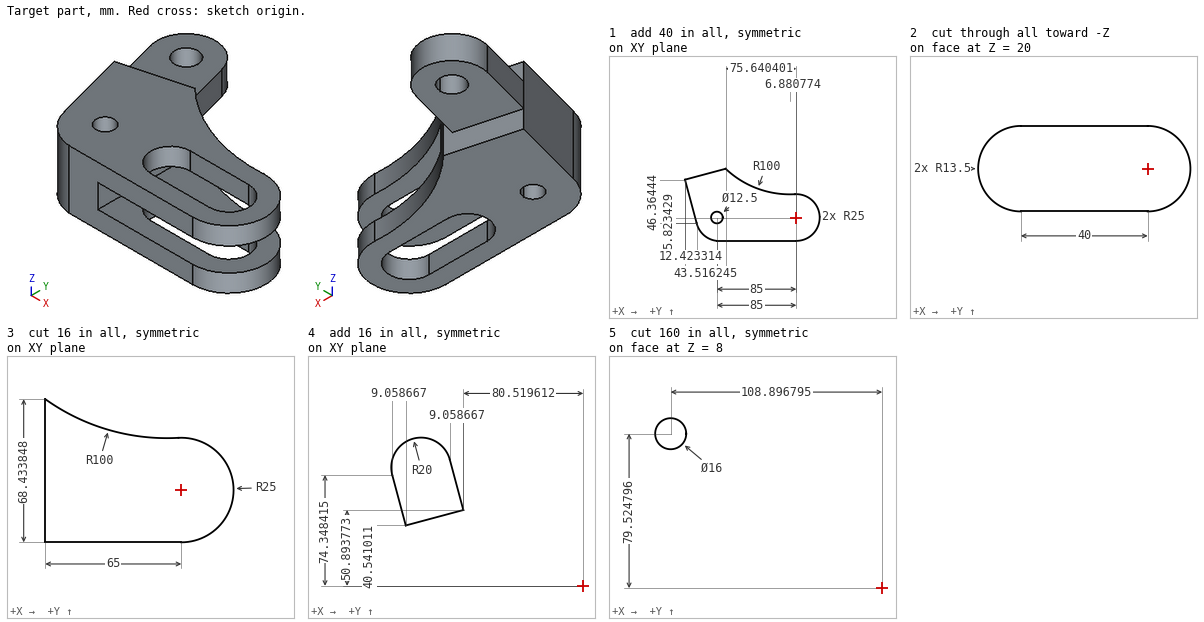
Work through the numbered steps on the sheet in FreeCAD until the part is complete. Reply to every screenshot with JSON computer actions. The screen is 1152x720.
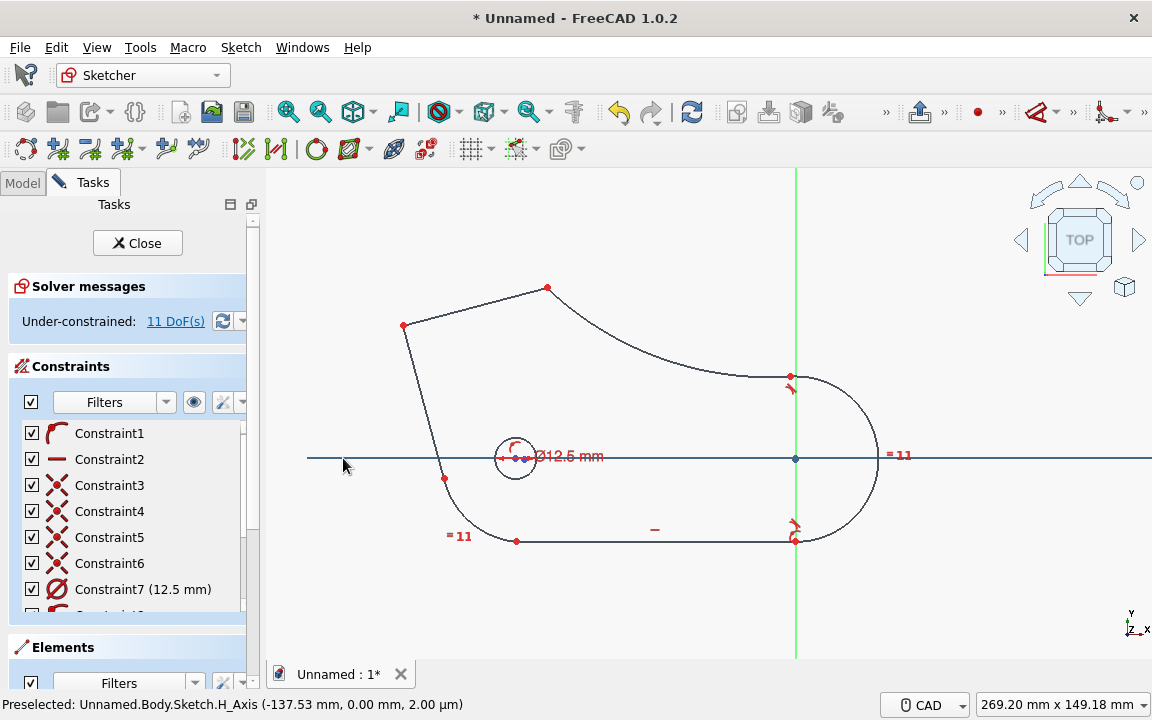
{"action": "key", "text": "c"}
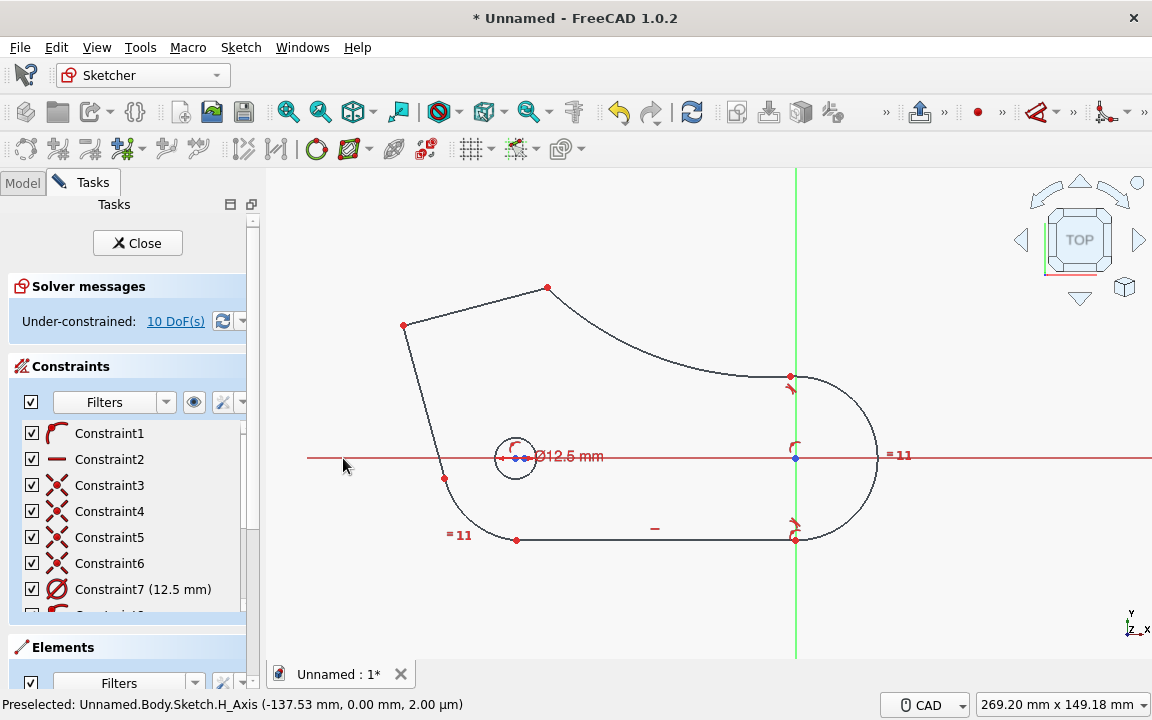
{"action": "left_click", "coordinate": [1036, 112]}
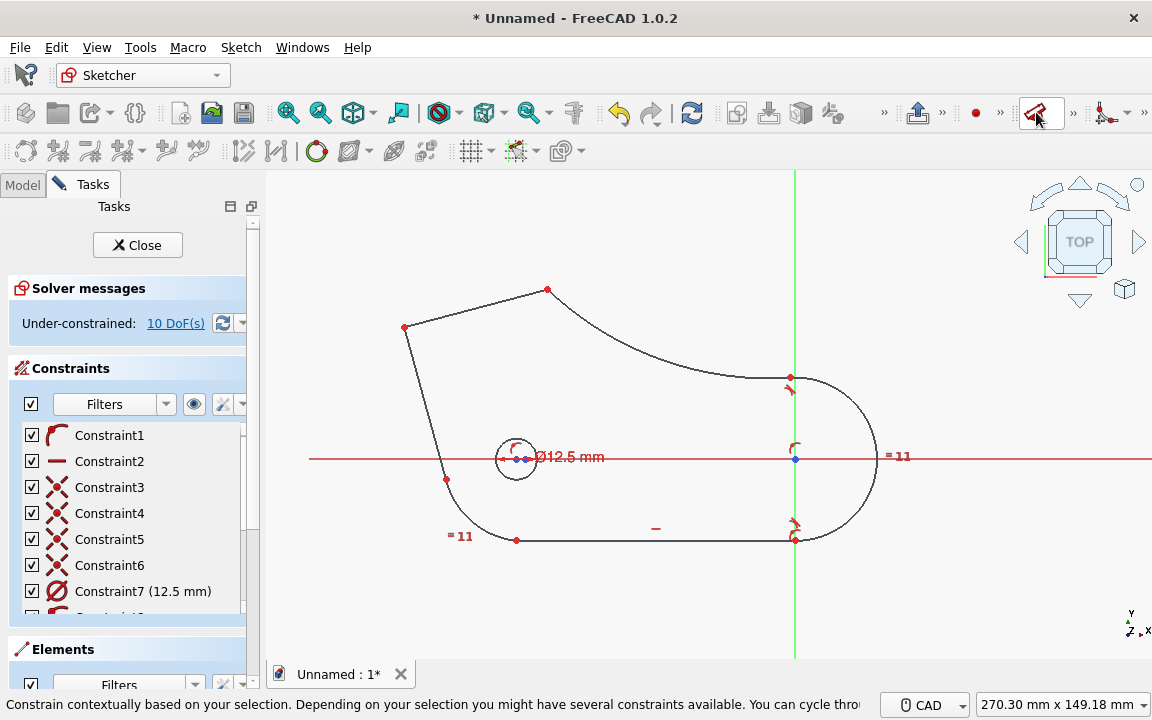
{"action": "left_click", "coordinate": [862, 506]}
{"action": "left_click", "coordinate": [888, 524]}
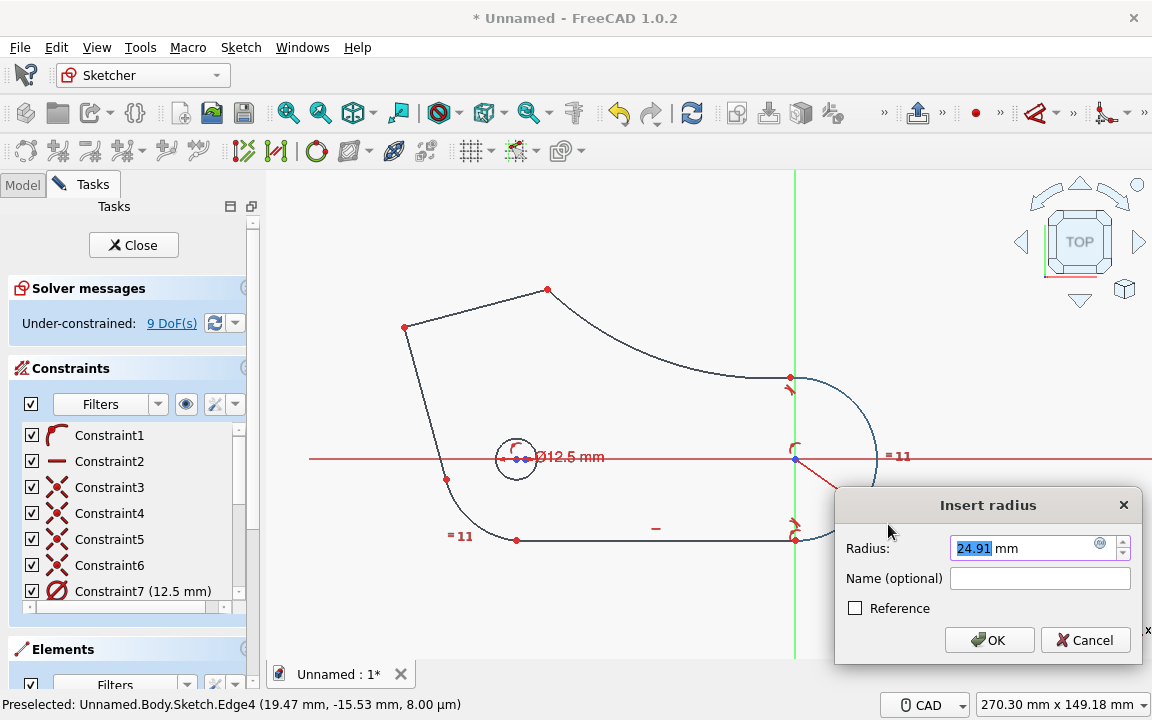
{"action": "type", "text": "25"}
{"action": "key", "text": "Return"}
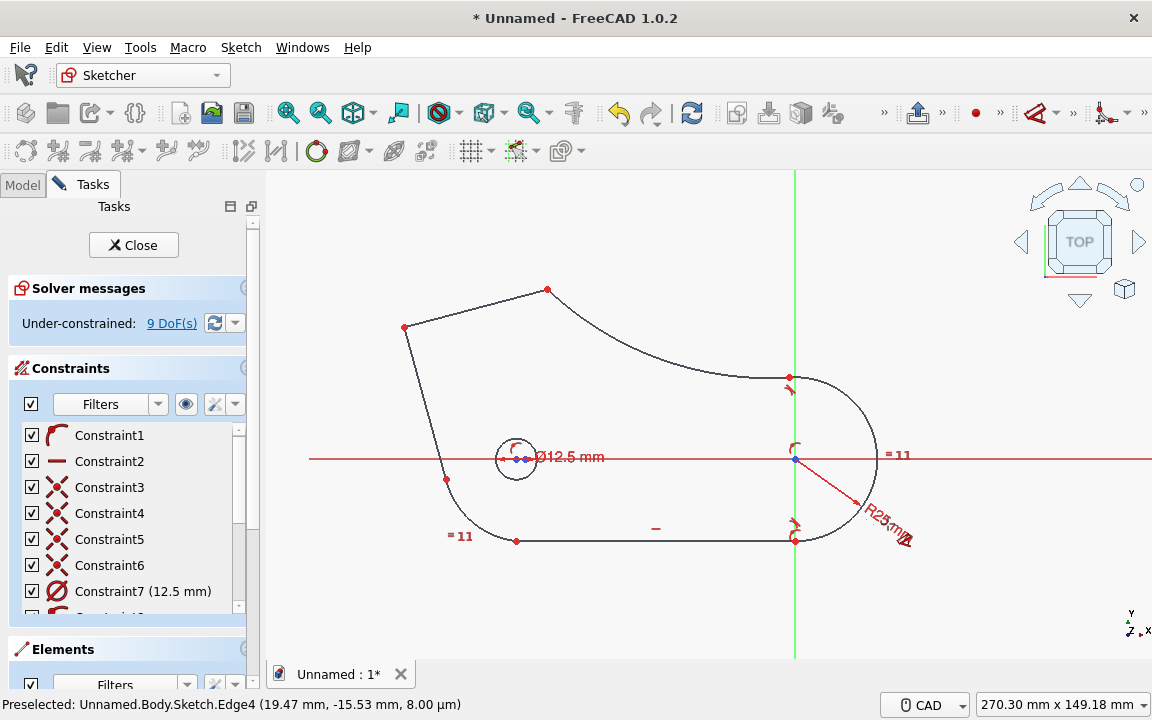
{"action": "left_click", "coordinate": [611, 337]}
{"action": "left_click", "coordinate": [595, 365]}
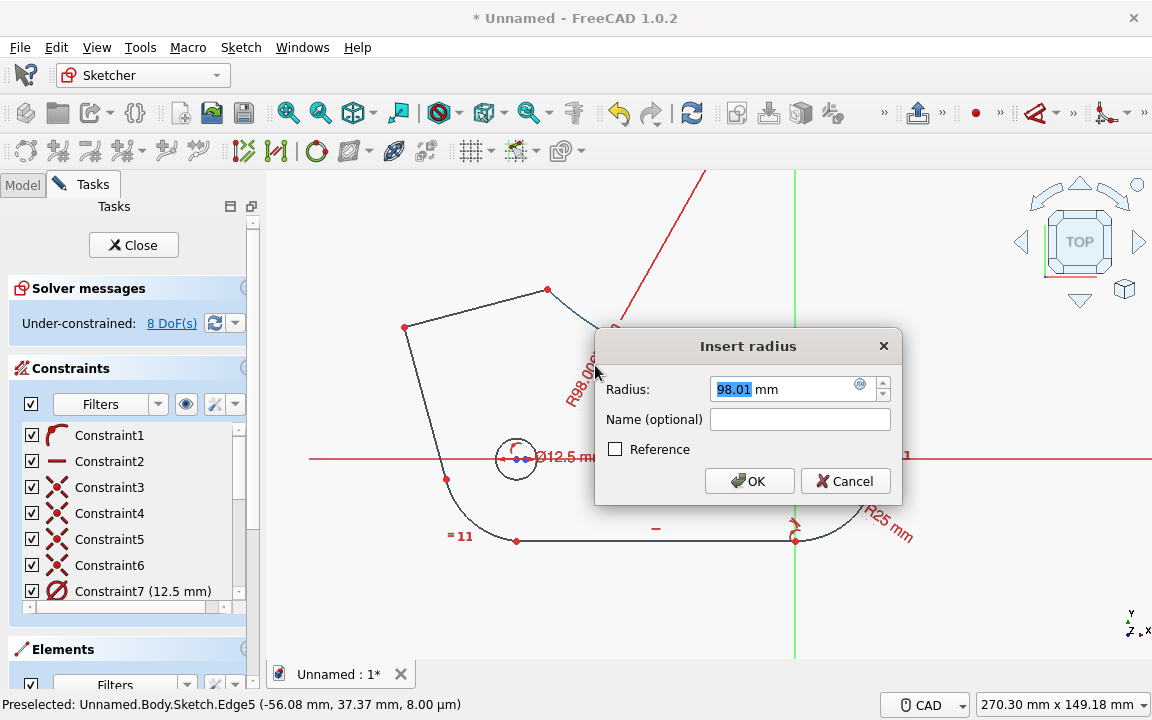
{"action": "type", "text": "100"}
{"action": "key", "text": "Return"}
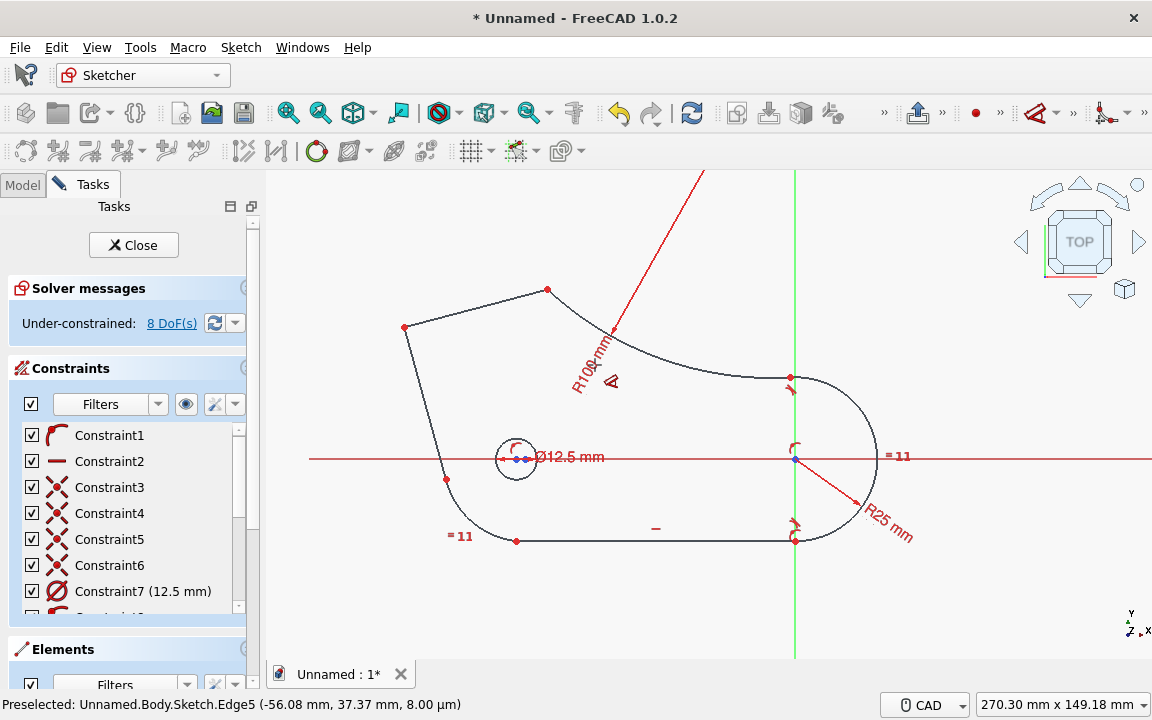
{"action": "left_click", "coordinate": [600, 541]}
{"action": "left_click", "coordinate": [656, 575]}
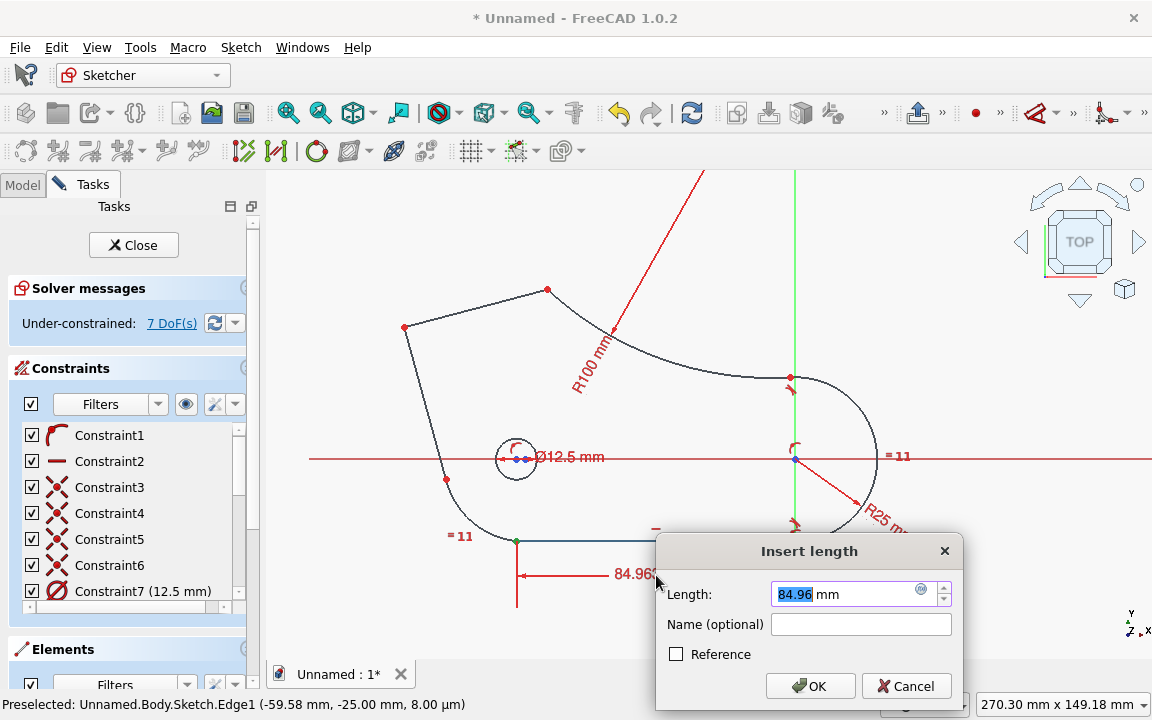
{"action": "type", "text": "85"}
{"action": "key", "text": "Return"}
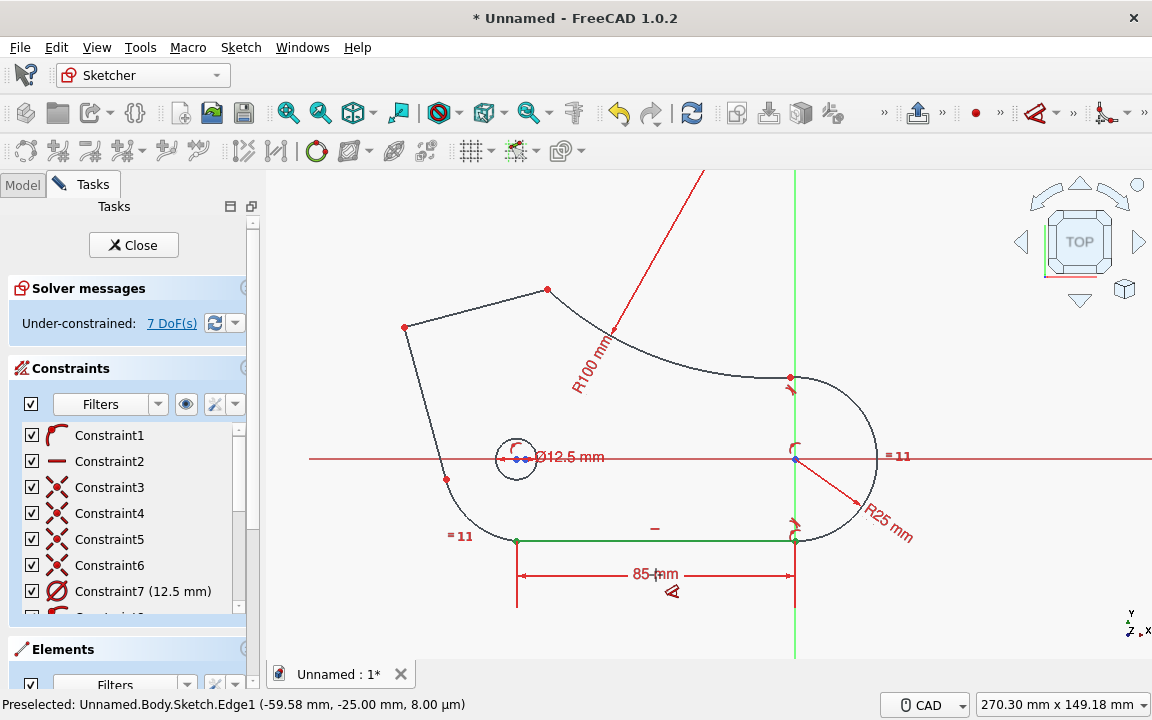
{"action": "scroll", "coordinate": [516, 459], "scroll_direction": "up", "scroll_amount": 2}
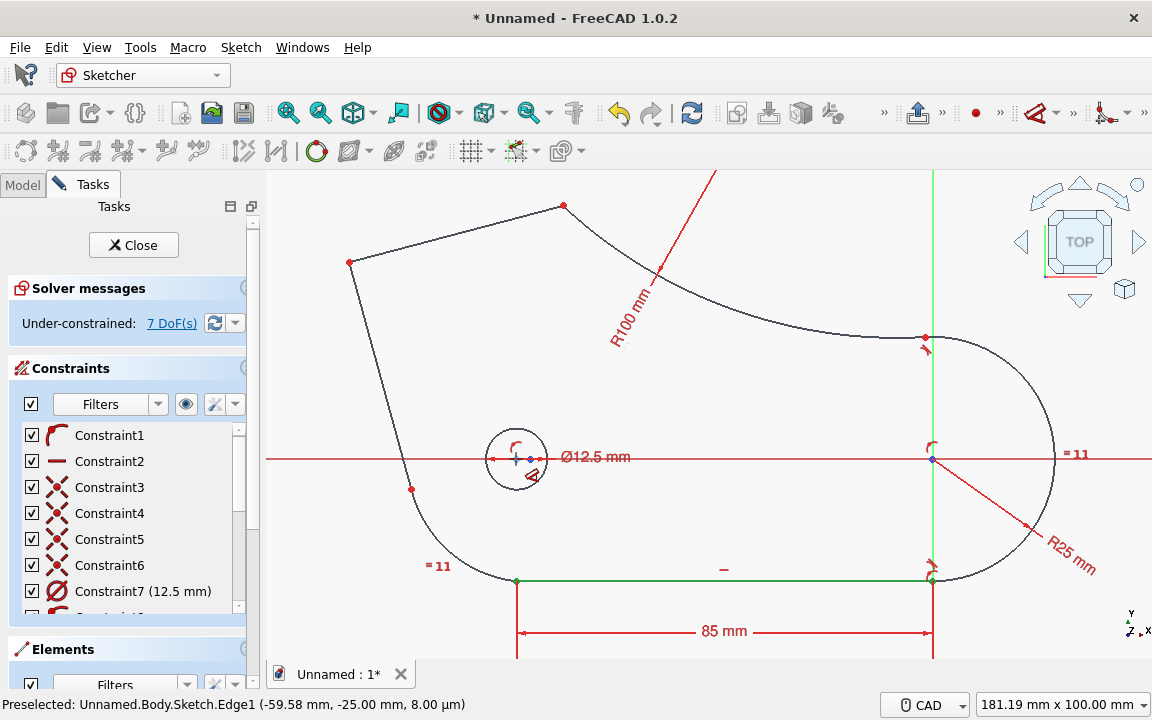
{"action": "left_click", "coordinate": [517, 459]}
{"action": "left_click", "coordinate": [725, 493]}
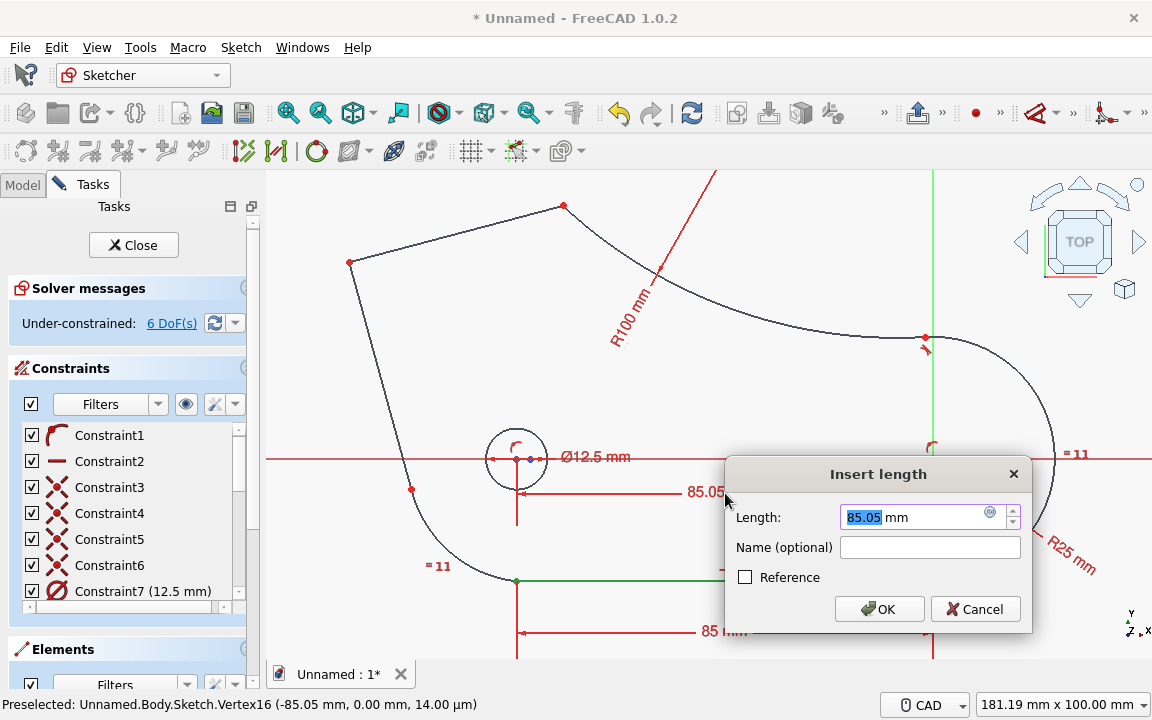
{"action": "type", "text": "85"}
{"action": "key", "text": "Return"}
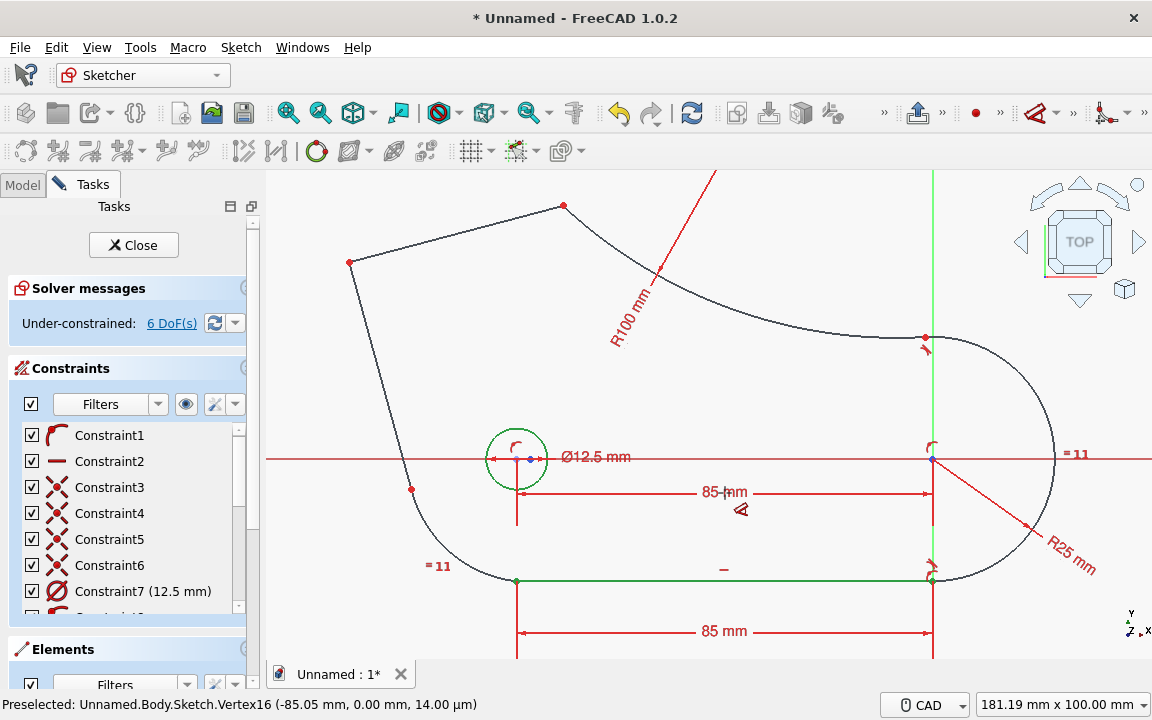
{"action": "scroll", "coordinate": [411, 490], "scroll_direction": "up", "scroll_amount": 2}